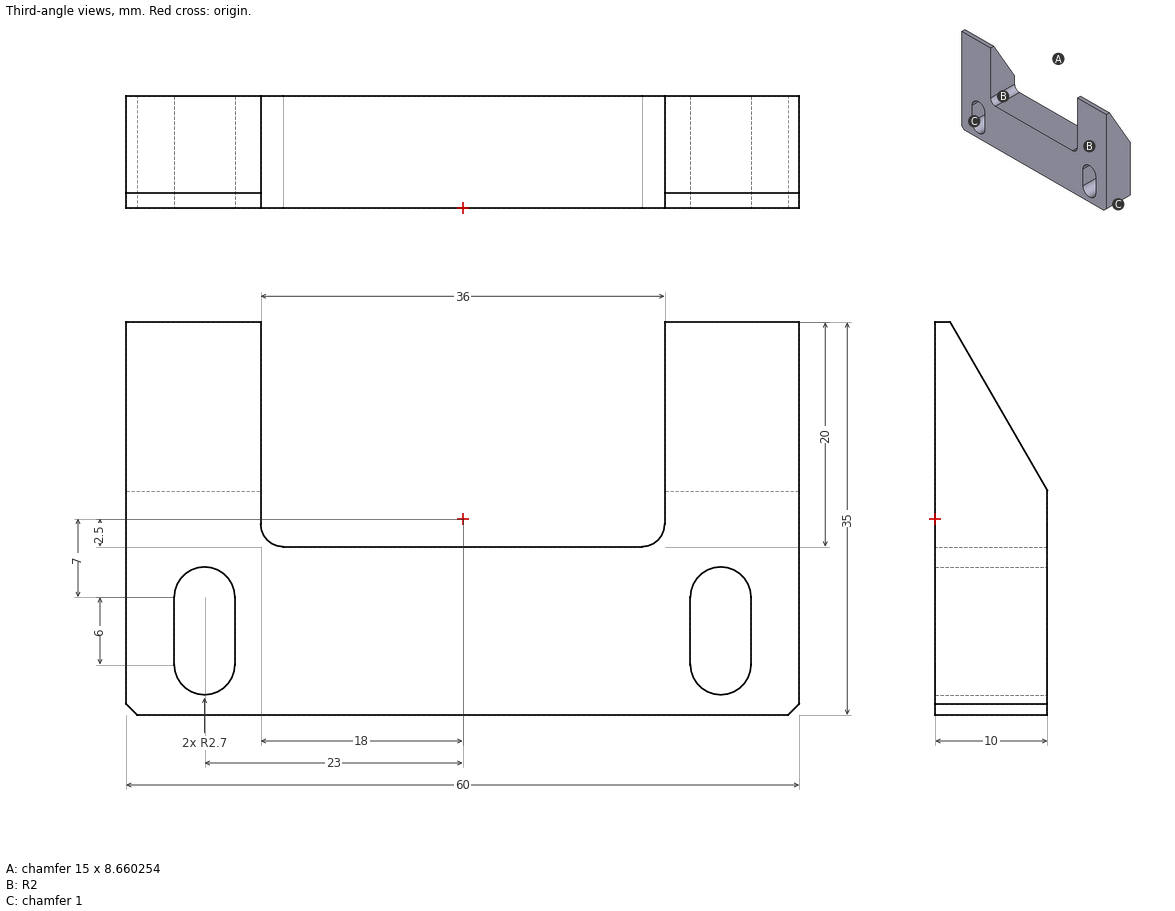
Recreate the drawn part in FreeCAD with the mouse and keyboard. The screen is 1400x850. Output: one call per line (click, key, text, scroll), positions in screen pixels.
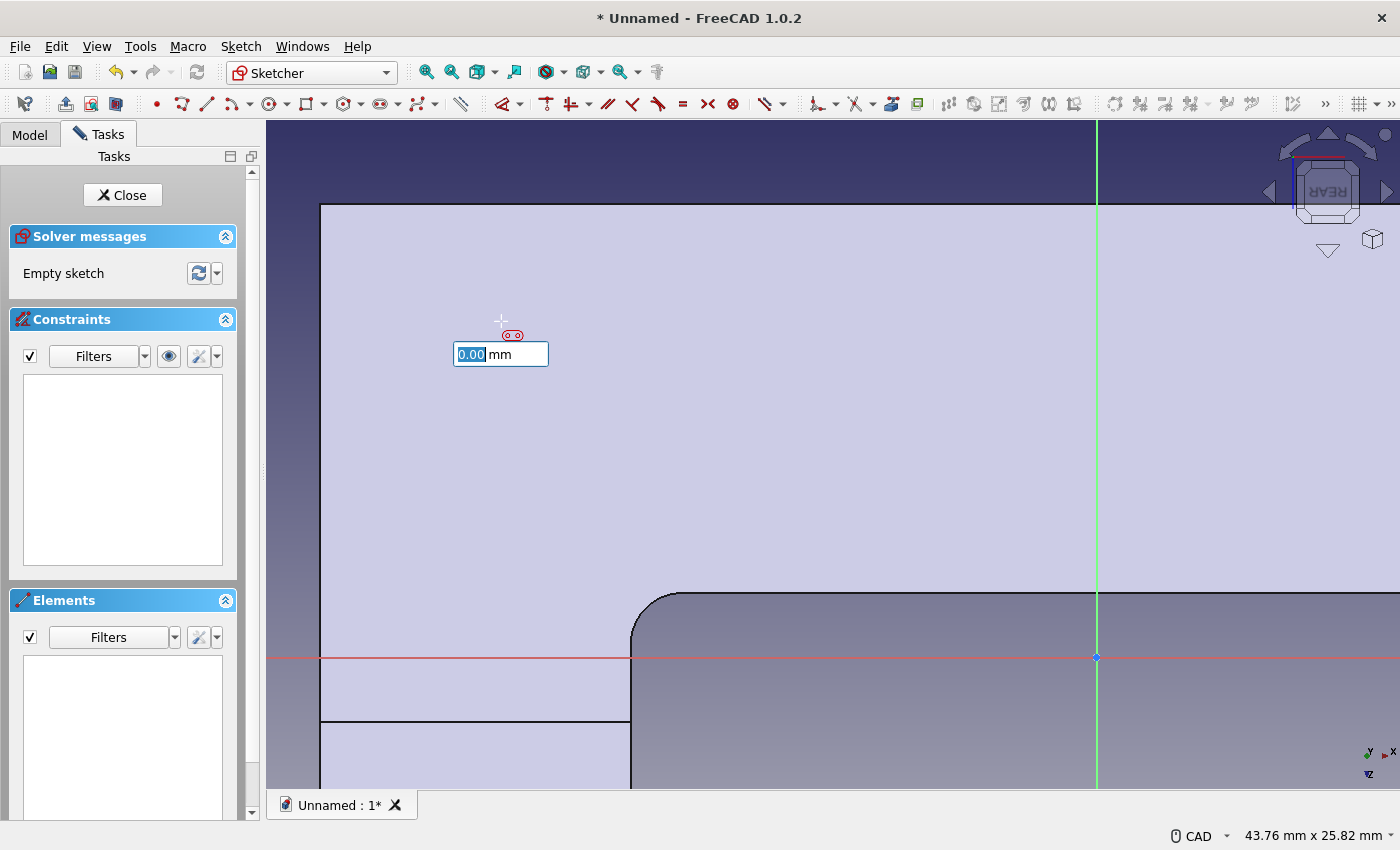
click(571, 398)
key(Escape)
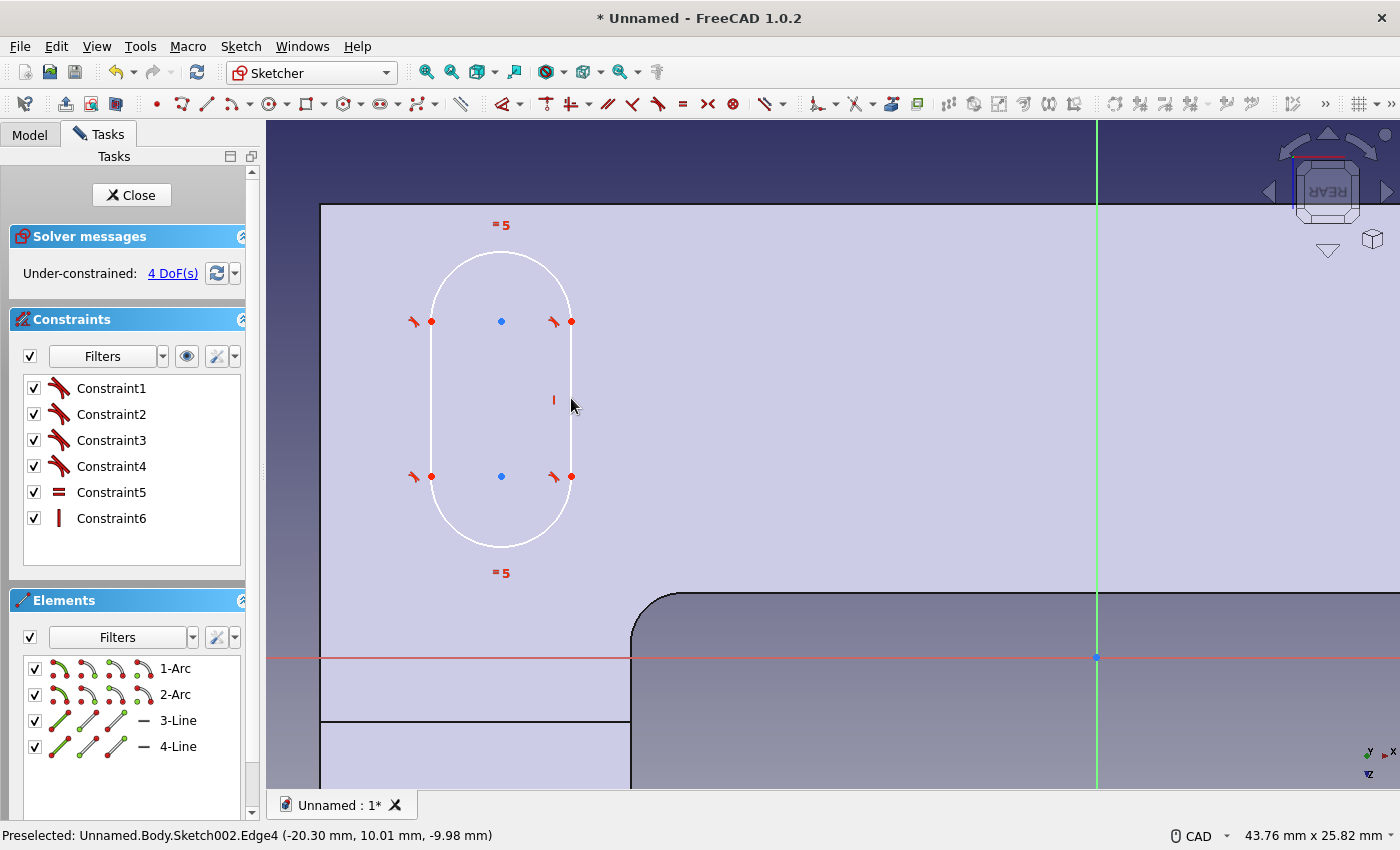
click(502, 104)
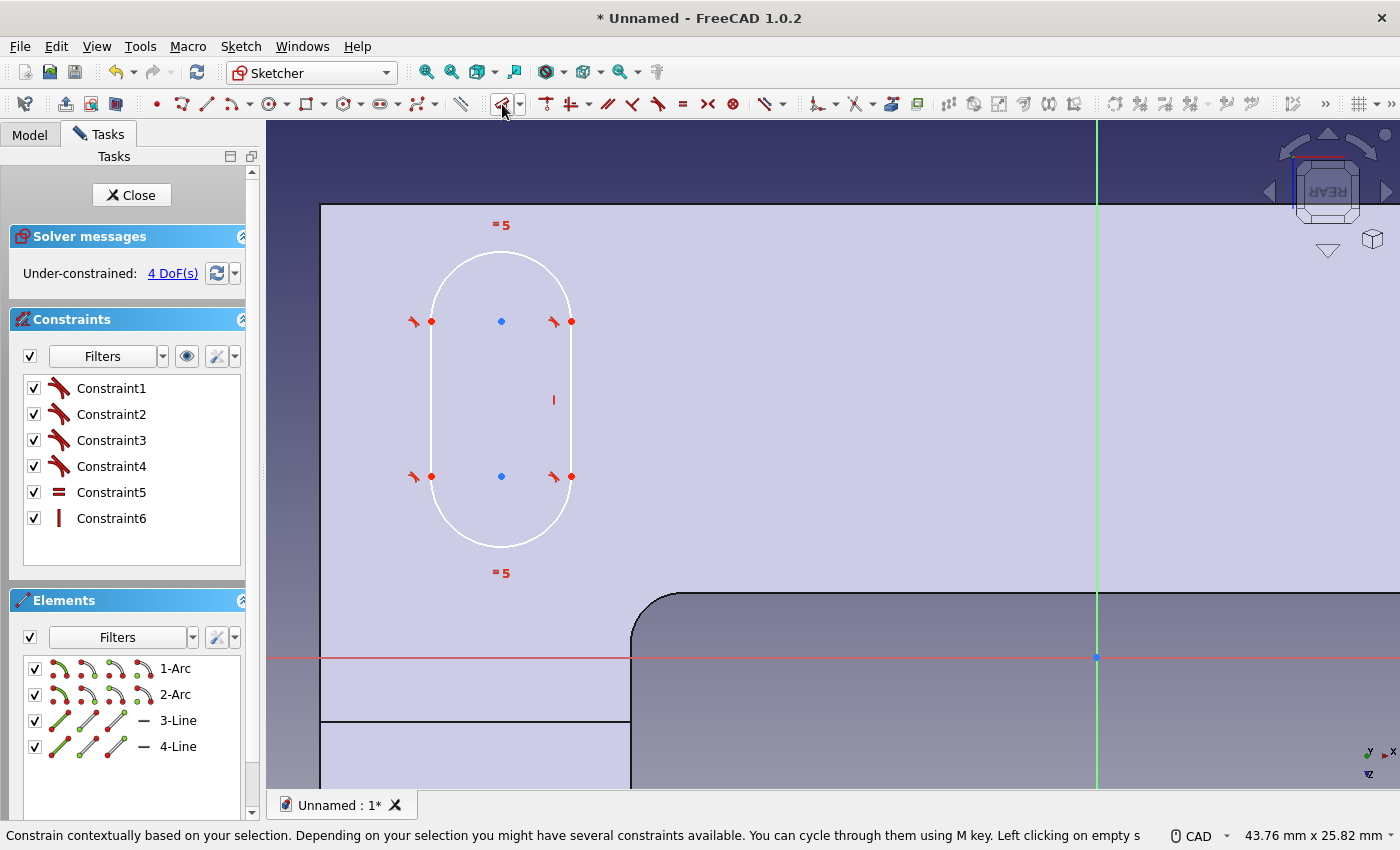
click(460, 534)
click(441, 560)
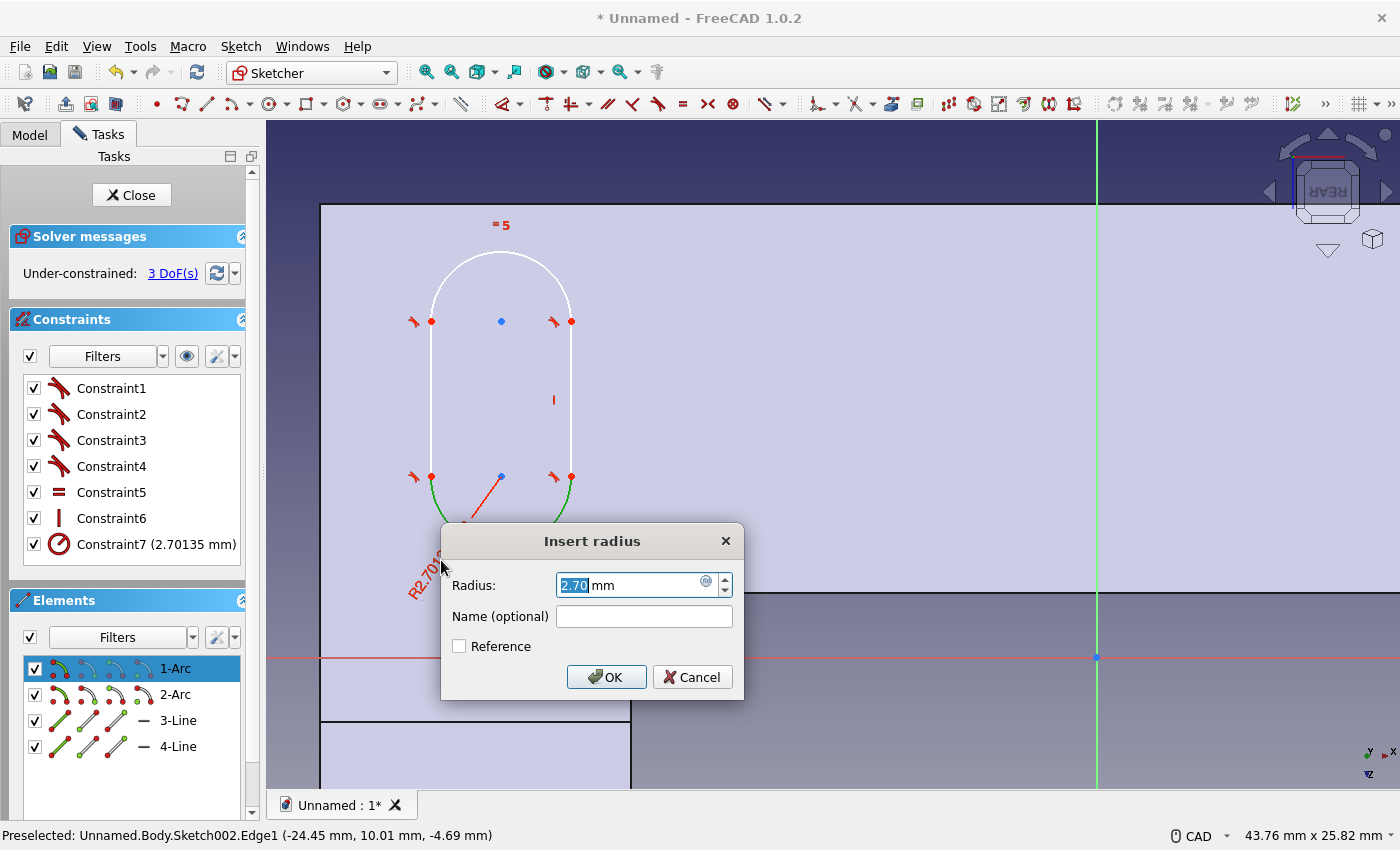
text(2.7)
key(Return)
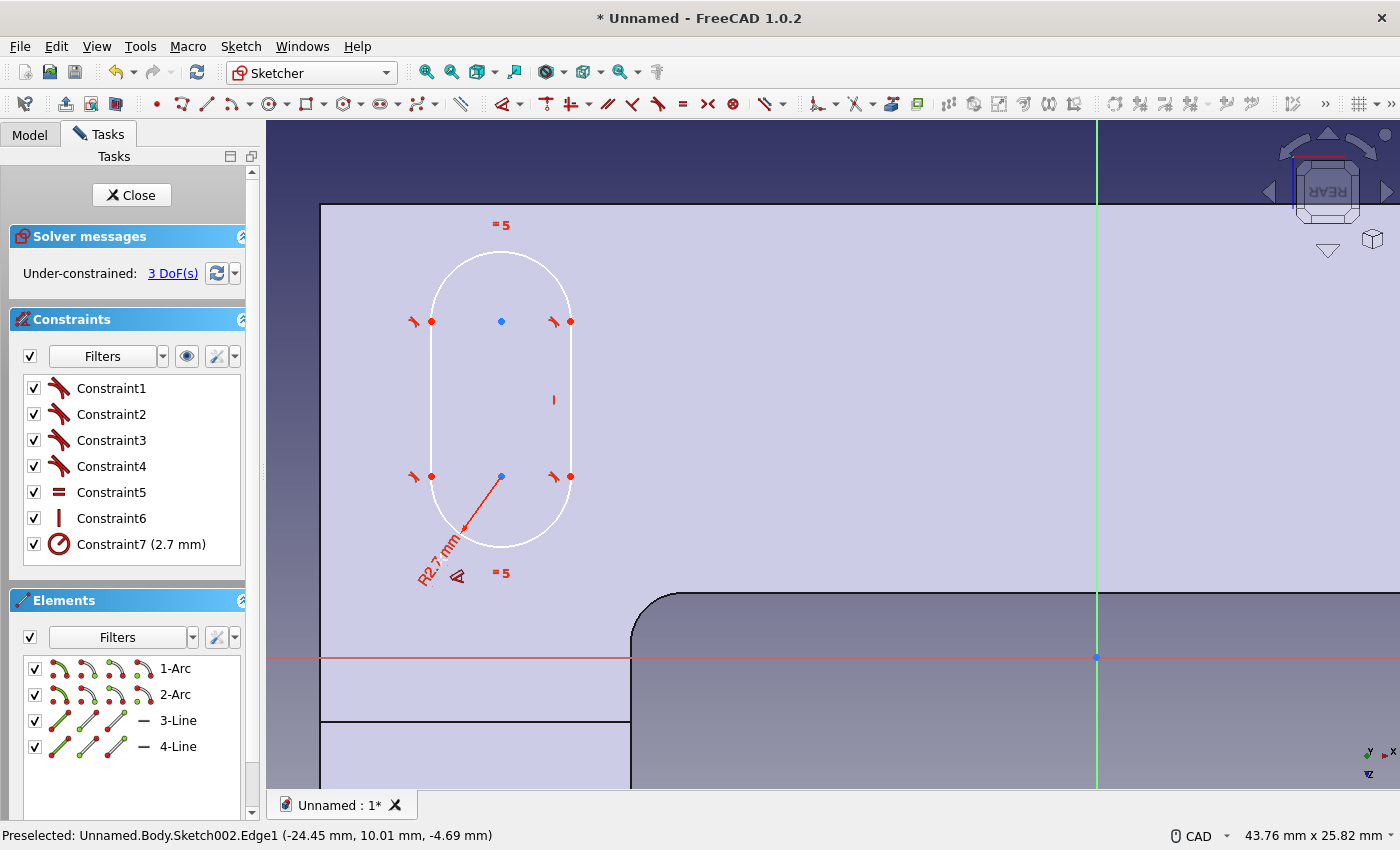
click(431, 431)
click(397, 399)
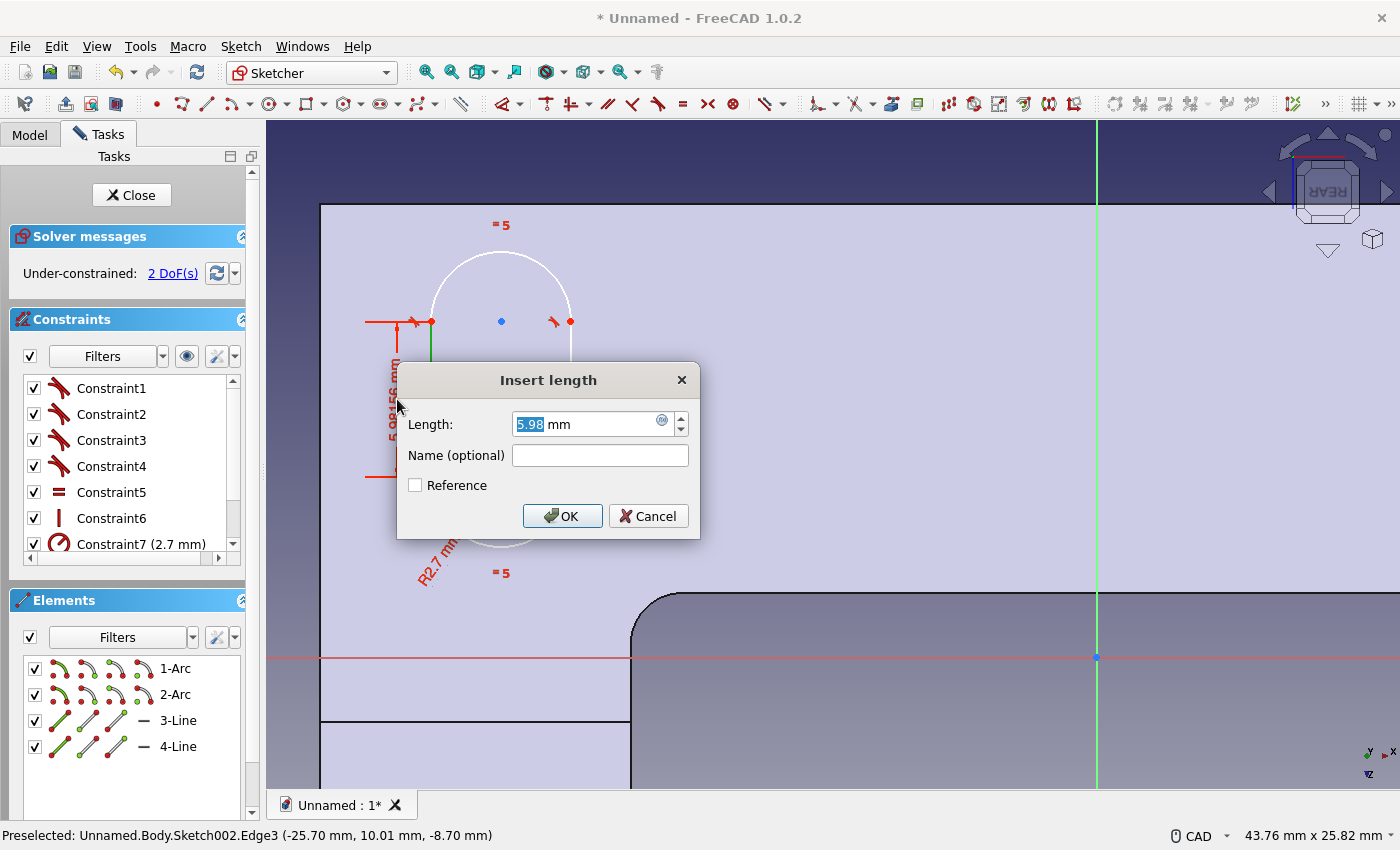
text(6)
key(Return)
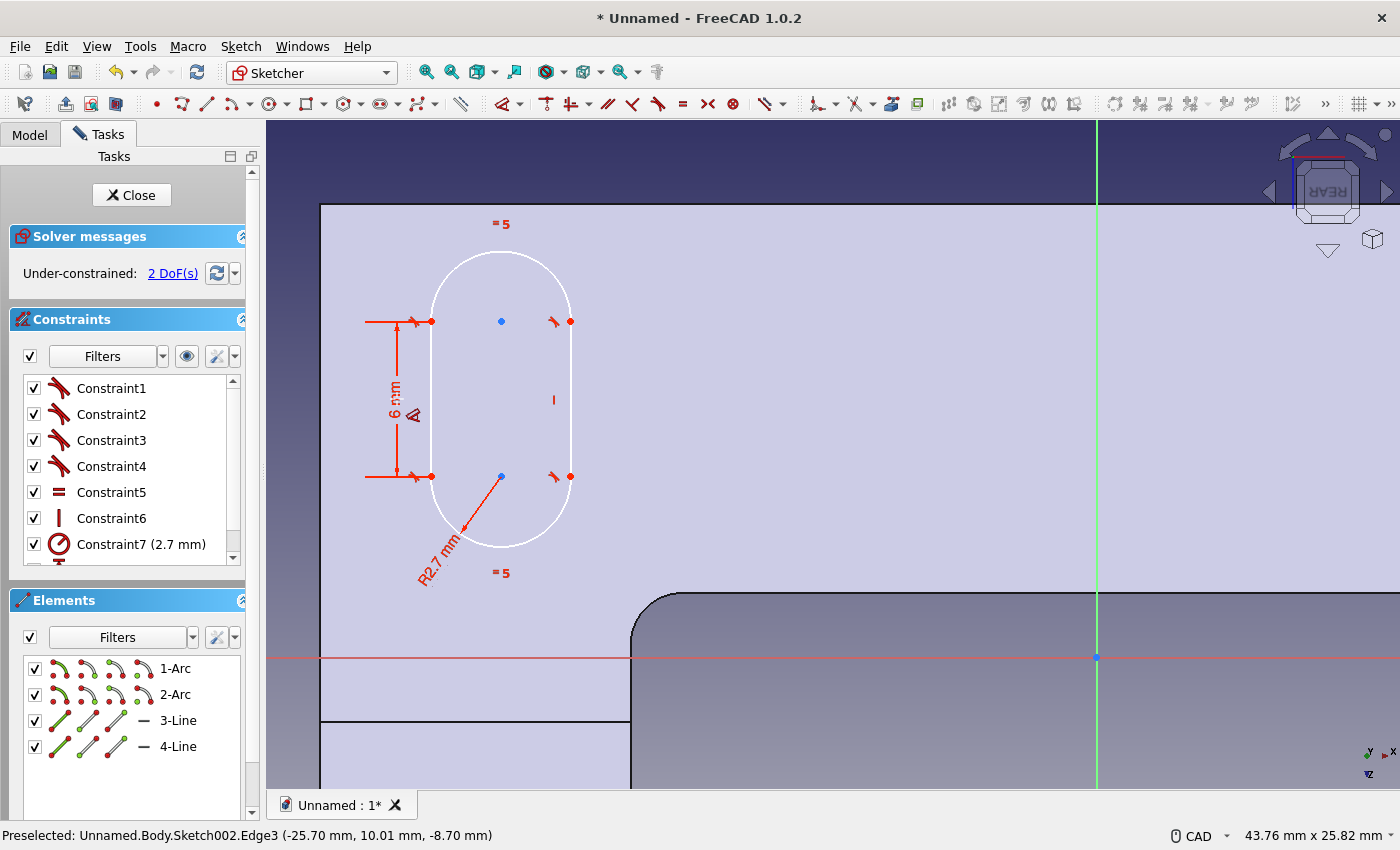
click(431, 477)
click(1131, 567)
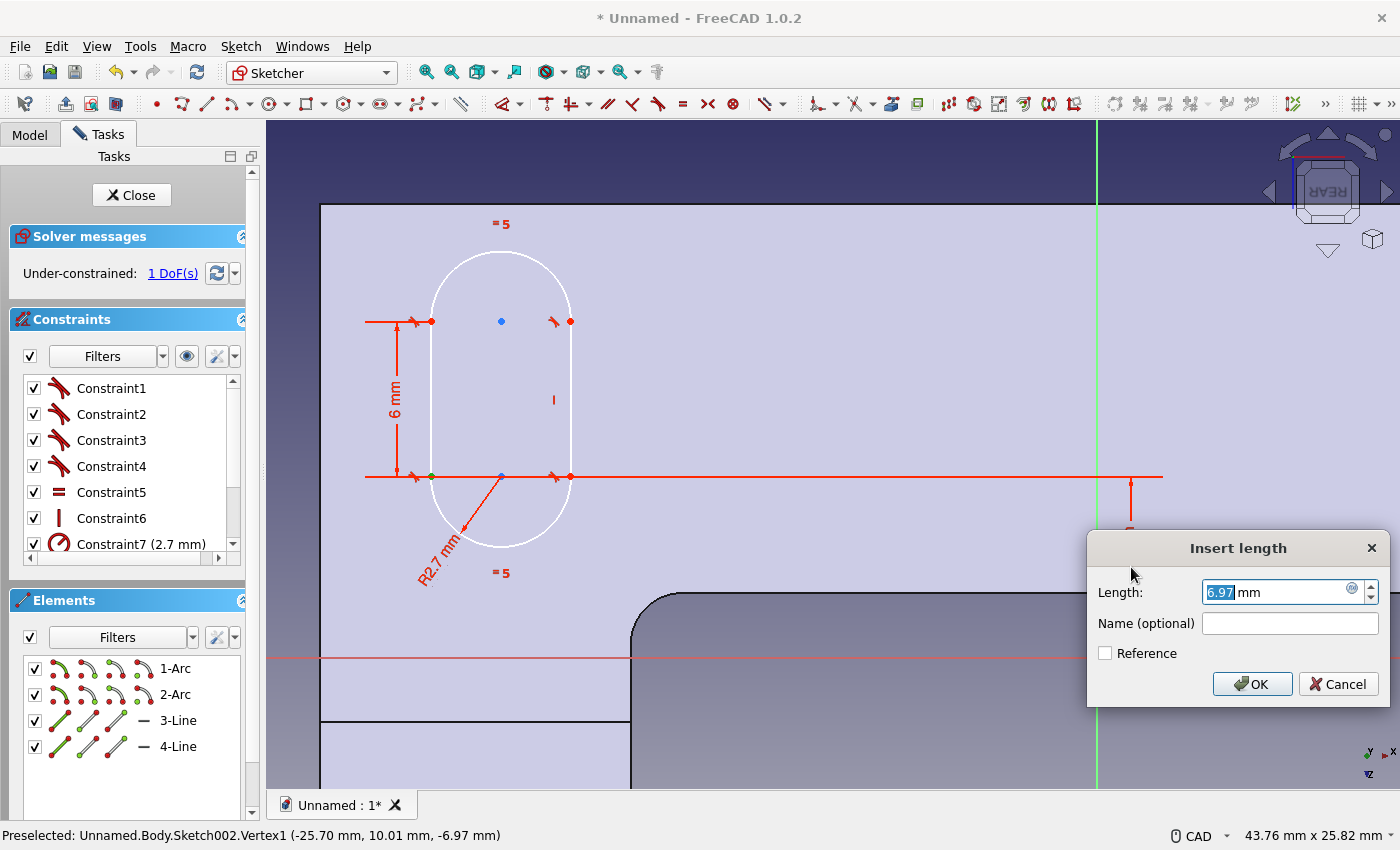
text(7)
key(Return)